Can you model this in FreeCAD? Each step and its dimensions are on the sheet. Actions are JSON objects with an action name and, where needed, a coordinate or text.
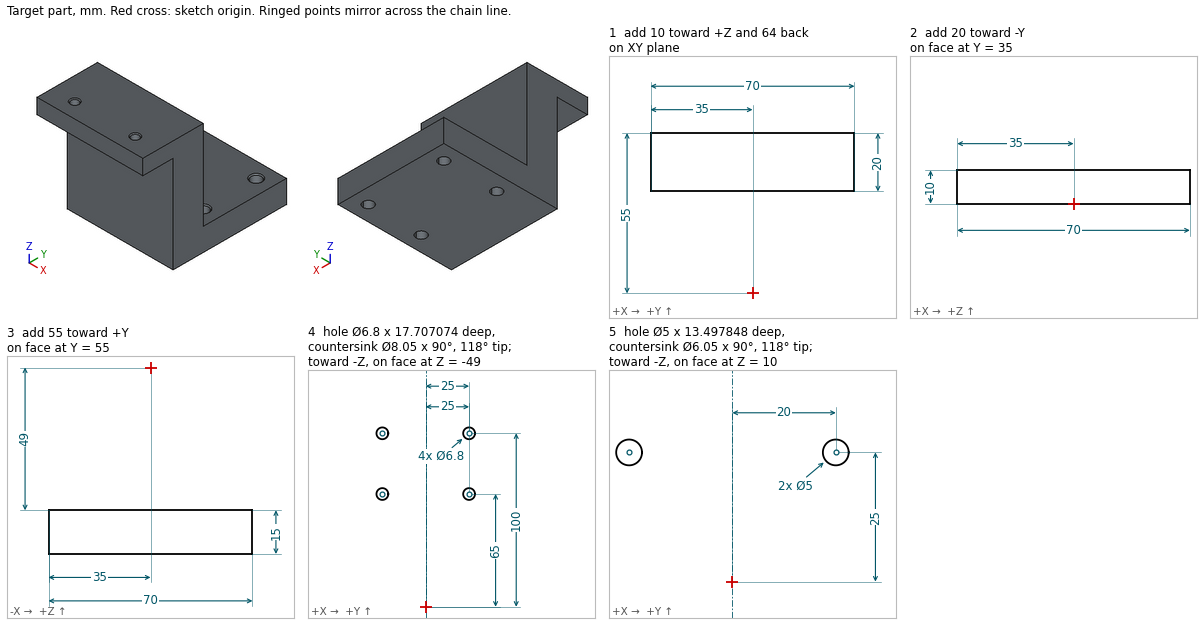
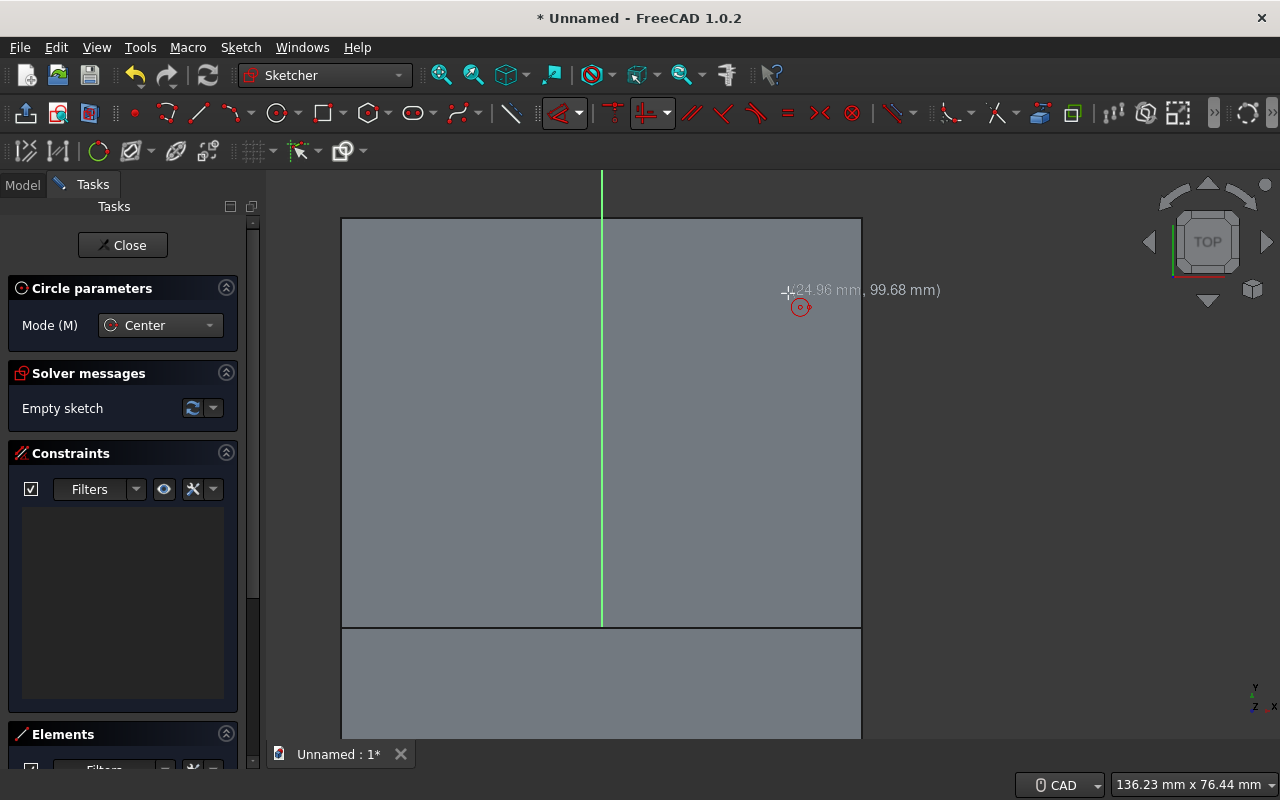
{"action": "left_click", "coordinate": [788, 293]}
{"action": "mouse_move", "coordinate": [806, 275]}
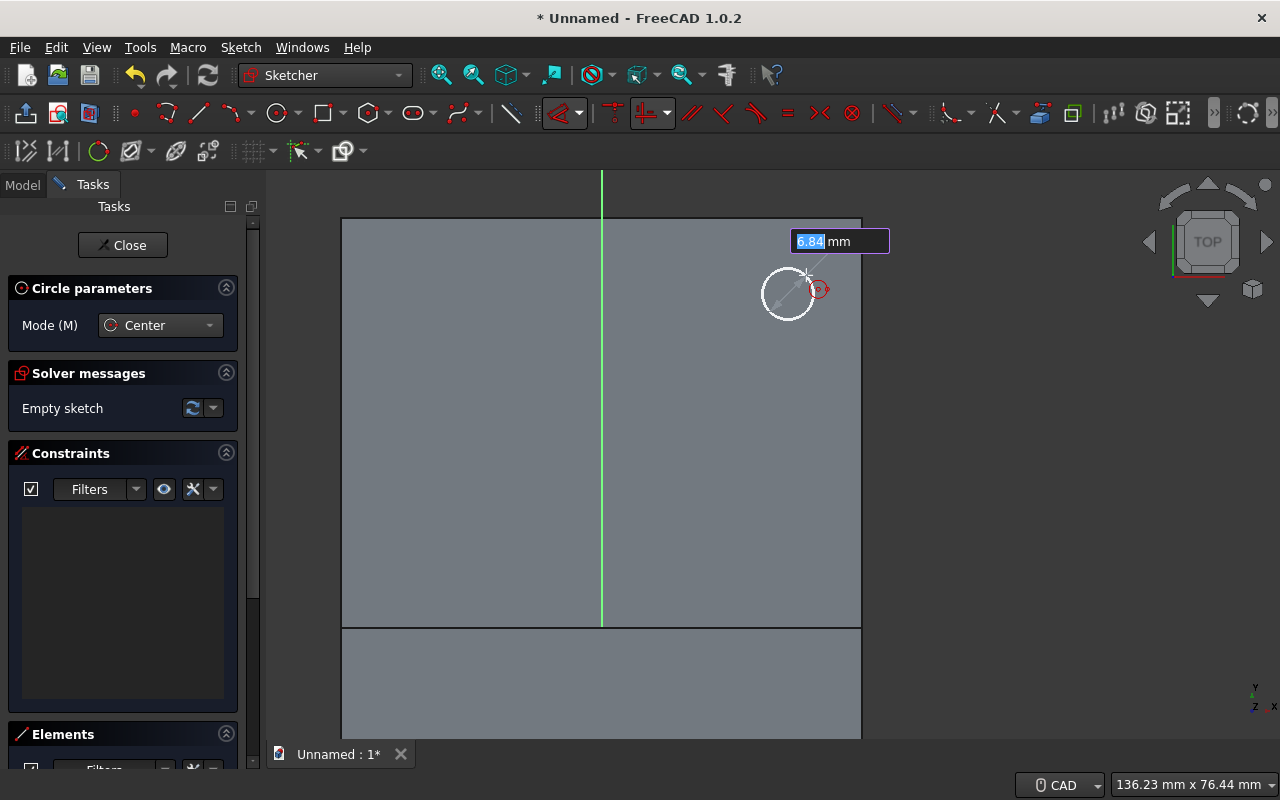
{"action": "type", "text": "6.8"}
{"action": "key", "text": "Return"}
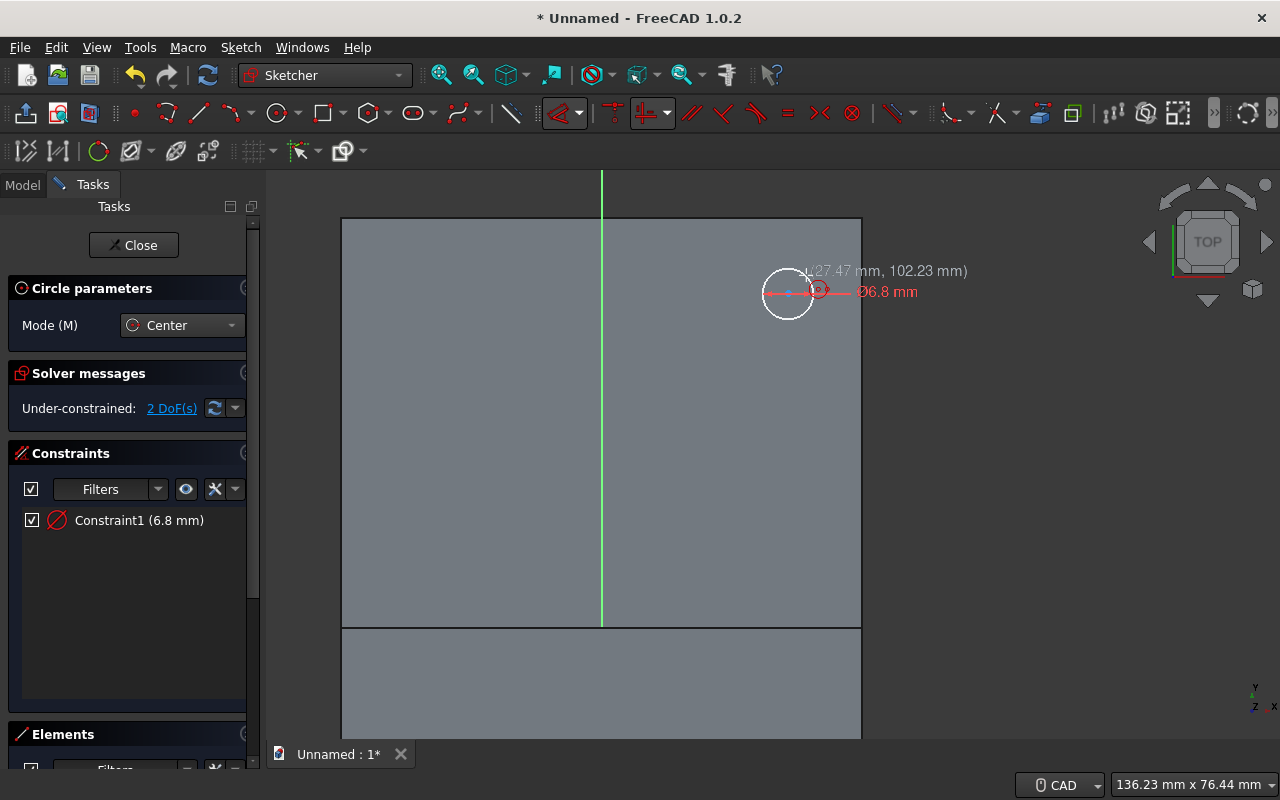
{"action": "left_click", "coordinate": [788, 553]}
{"action": "mouse_move", "coordinate": [806, 535]}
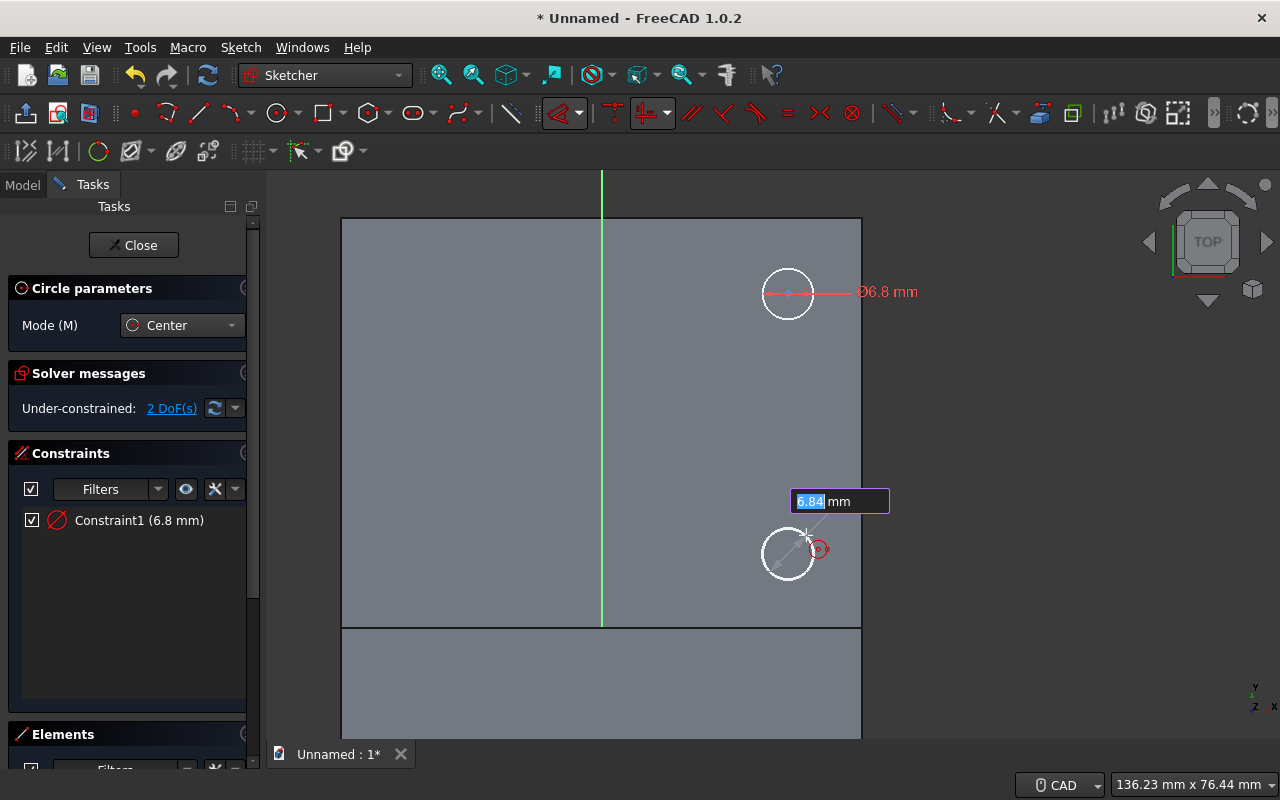
{"action": "type", "text": "6.8"}
{"action": "key", "text": "Return"}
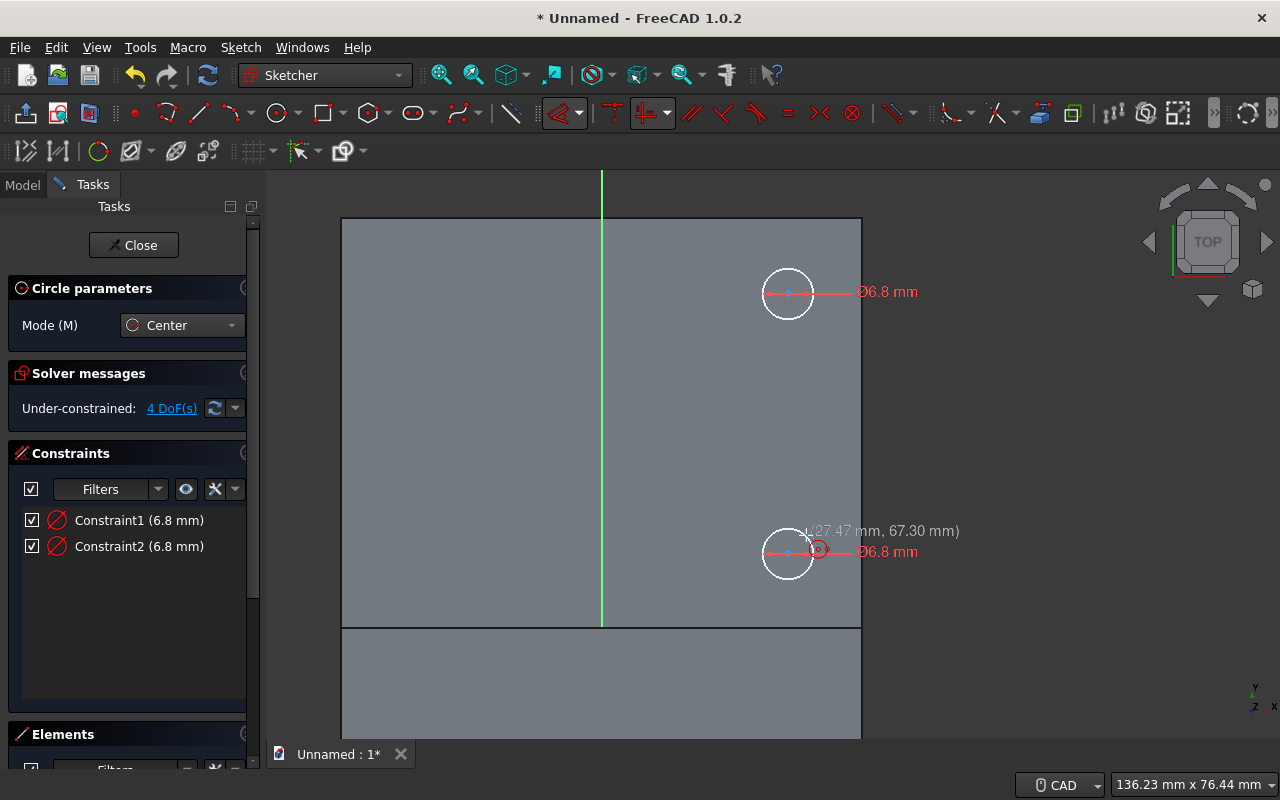
{"action": "left_click", "coordinate": [415, 553]}
{"action": "mouse_move", "coordinate": [433, 535]}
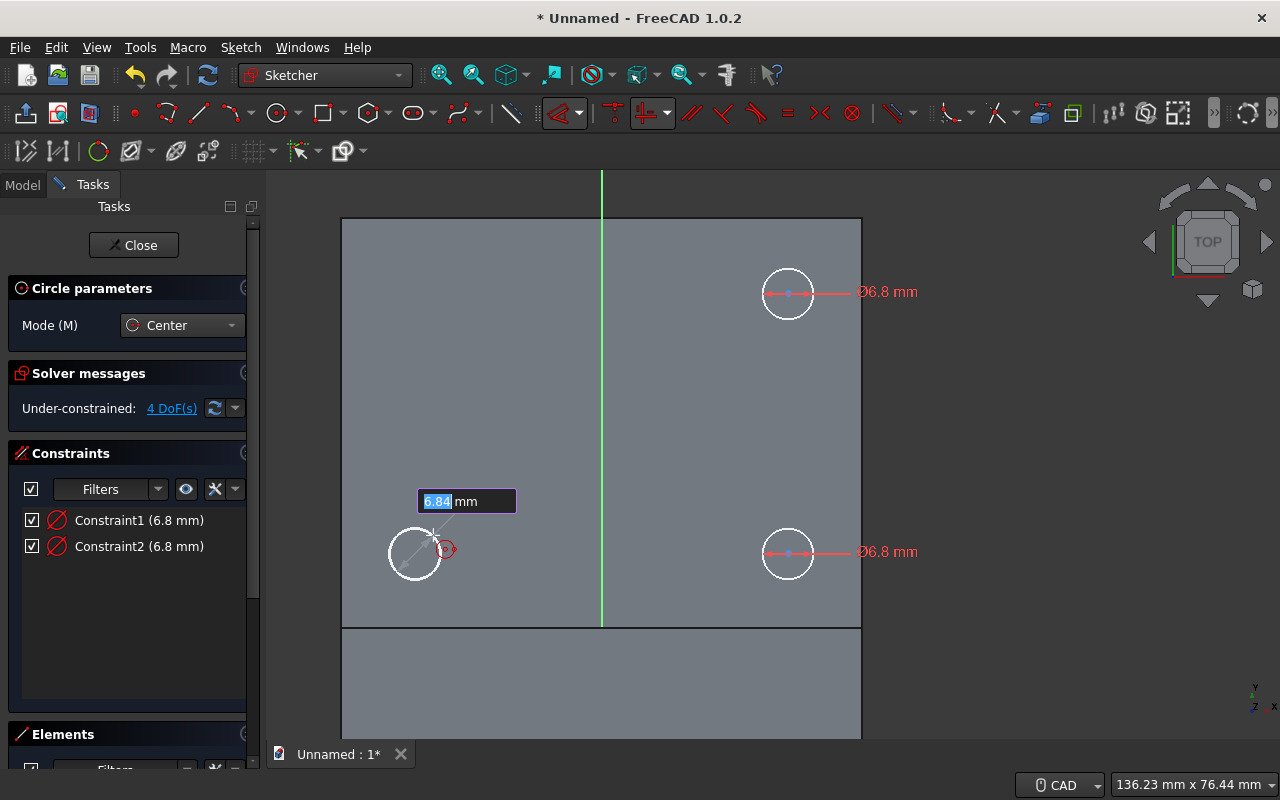
{"action": "type", "text": "6.8"}
{"action": "key", "text": "Return"}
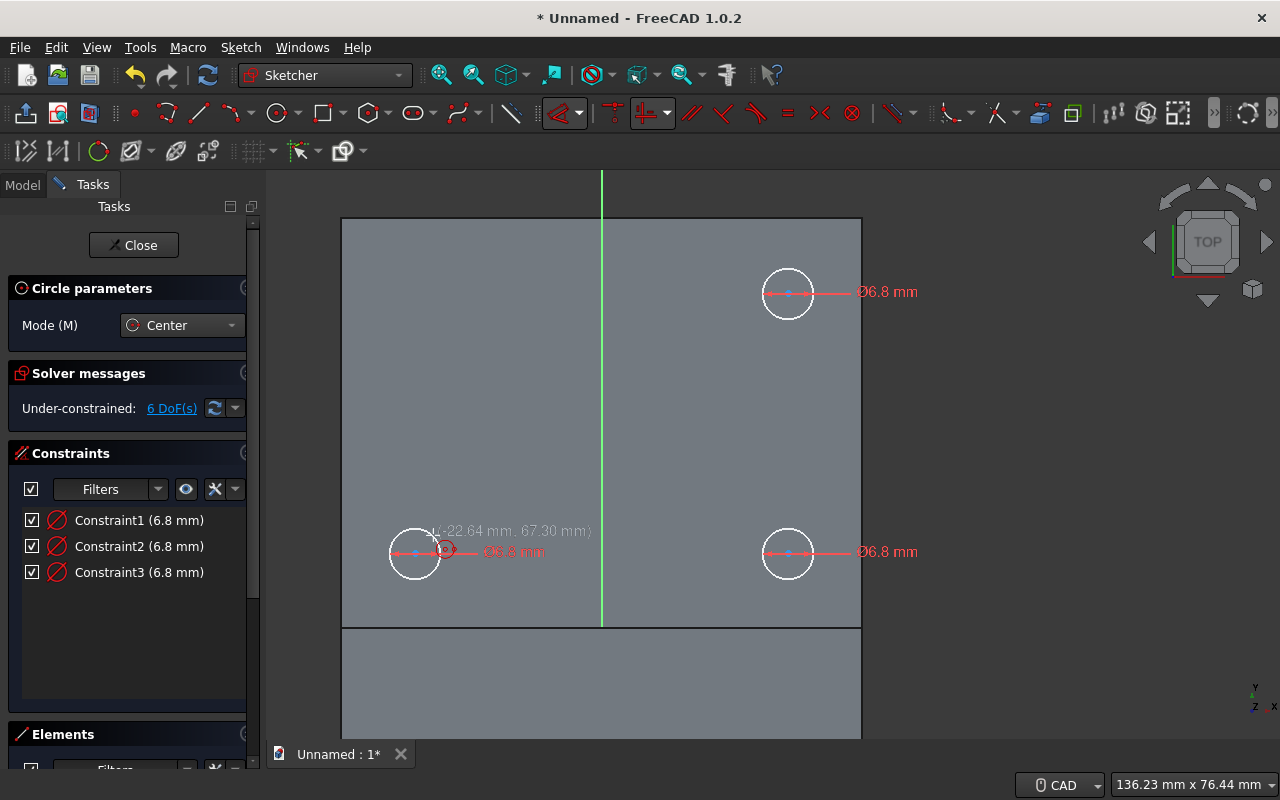
{"action": "left_click", "coordinate": [415, 293]}
{"action": "mouse_move", "coordinate": [433, 275]}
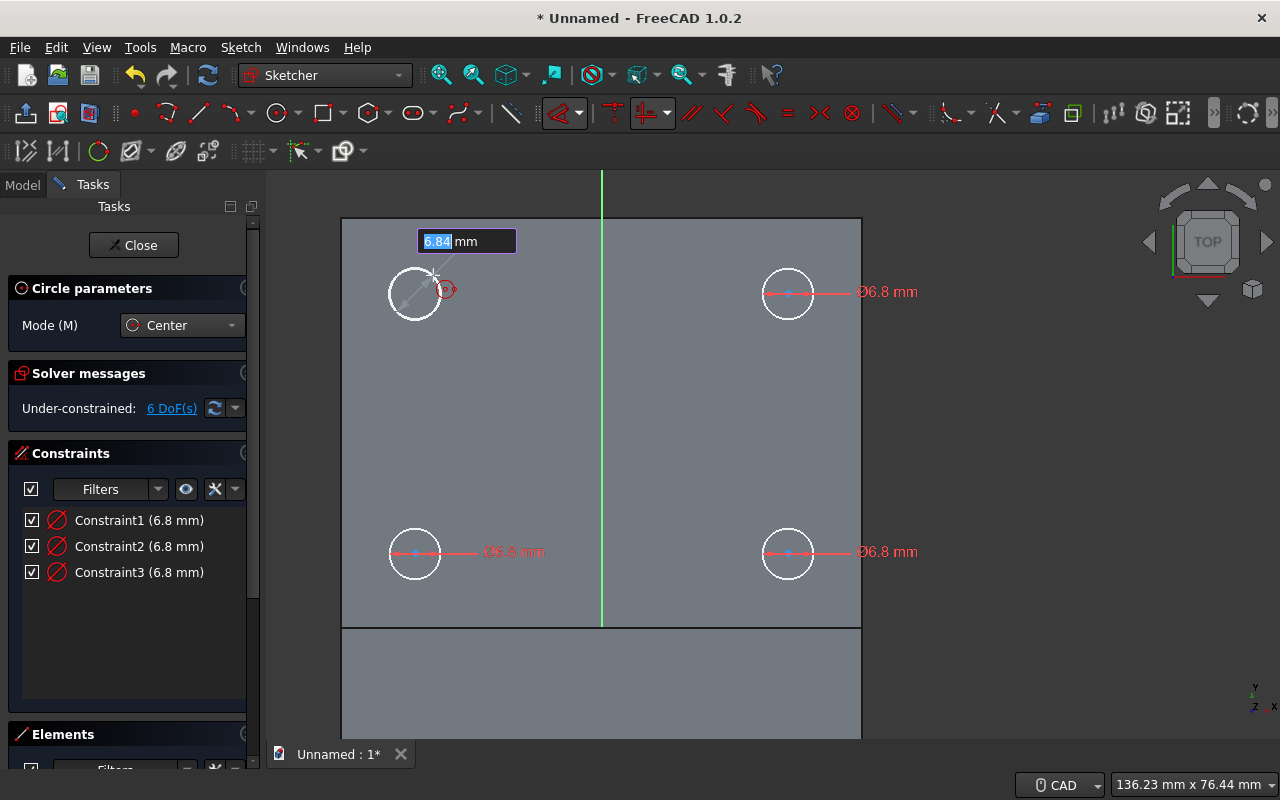
{"action": "type", "text": "6.8"}
{"action": "key", "text": "Return"}
{"action": "key", "text": "Escape"}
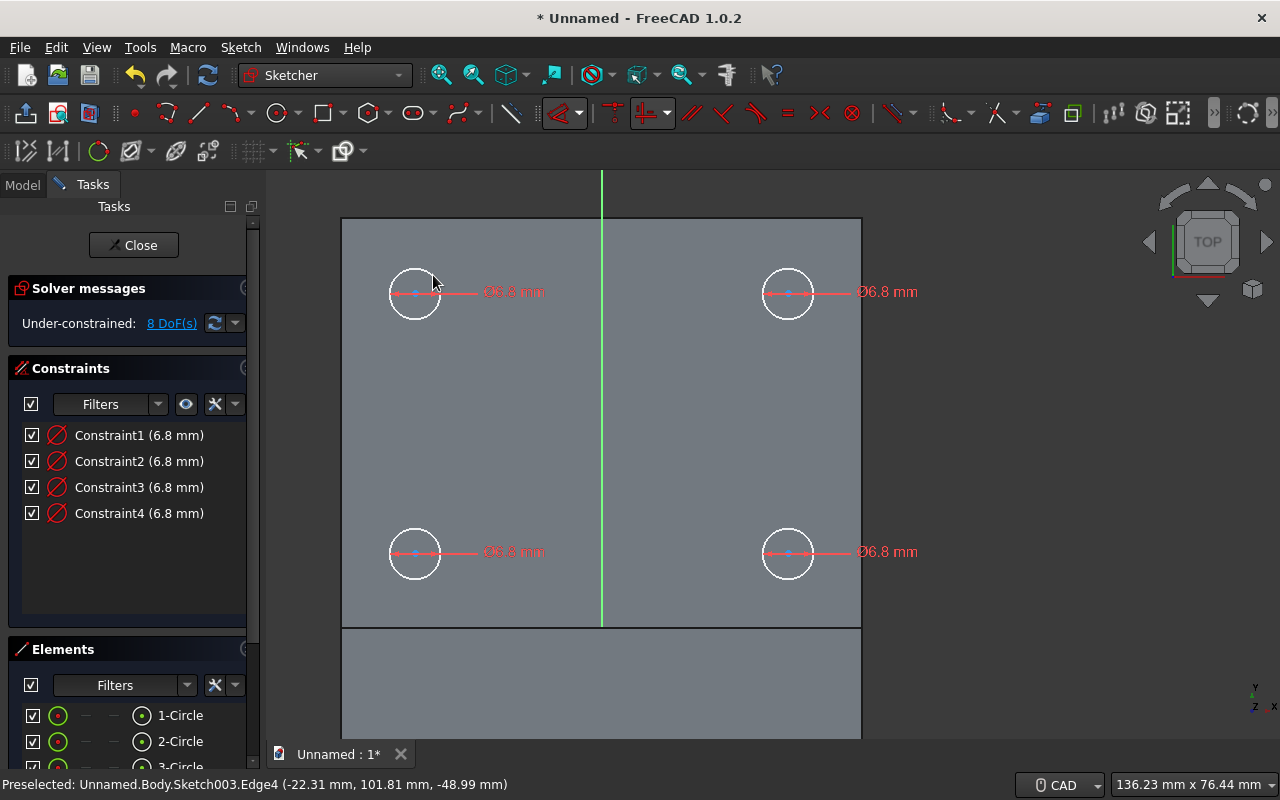
{"action": "left_click", "coordinate": [788, 554]}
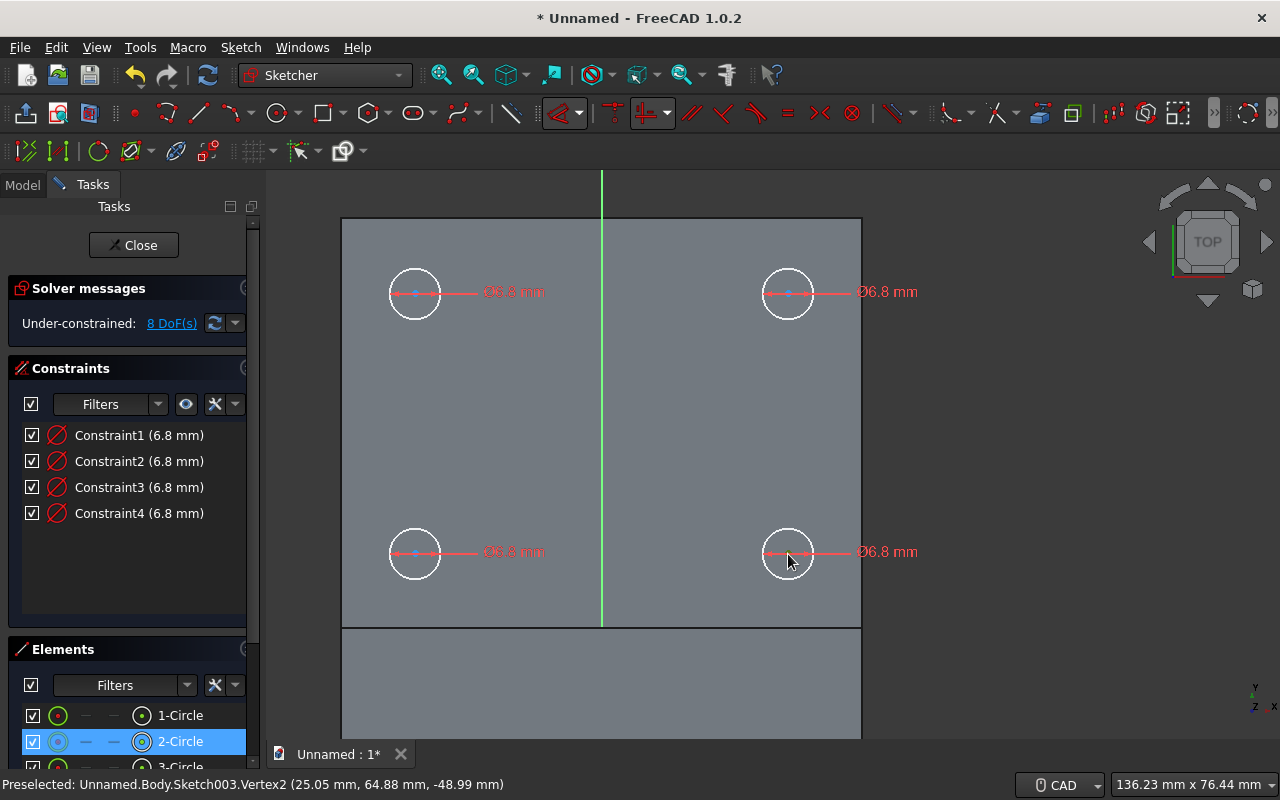
{"action": "left_click", "coordinate": [415, 554]}